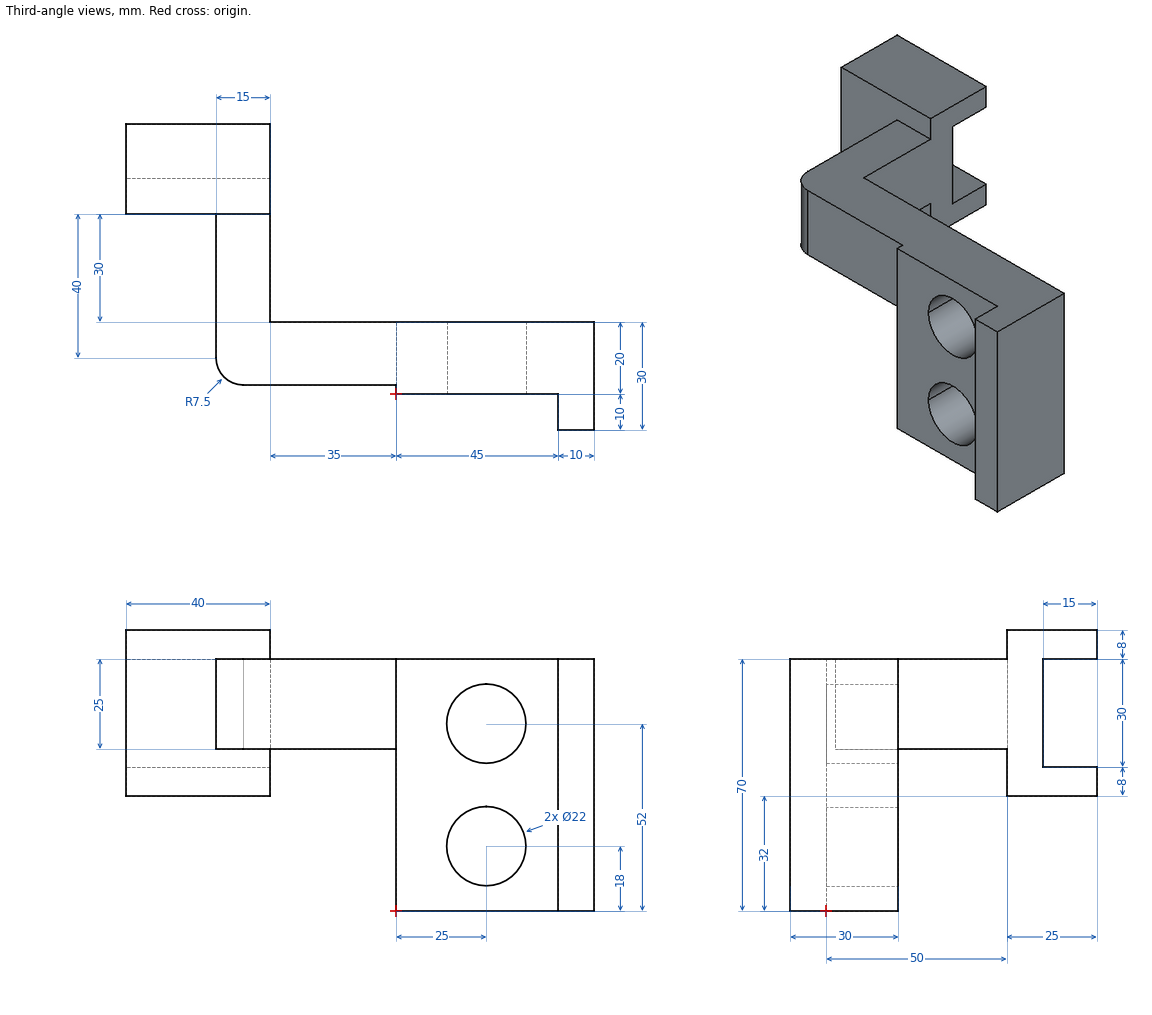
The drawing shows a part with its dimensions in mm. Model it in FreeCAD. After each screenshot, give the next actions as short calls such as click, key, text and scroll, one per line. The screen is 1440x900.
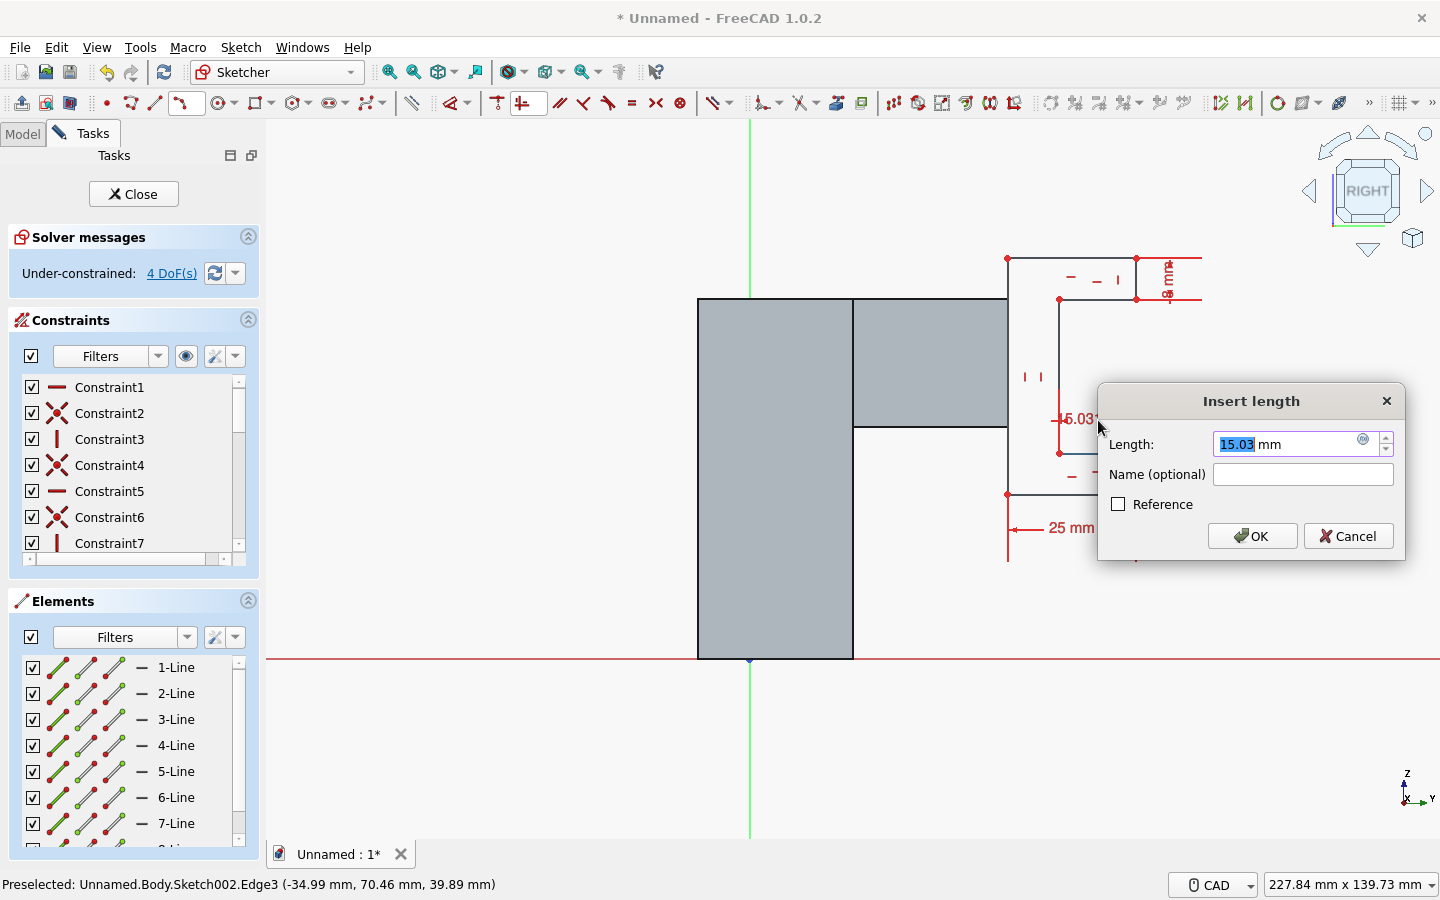
text(15)
key(Return)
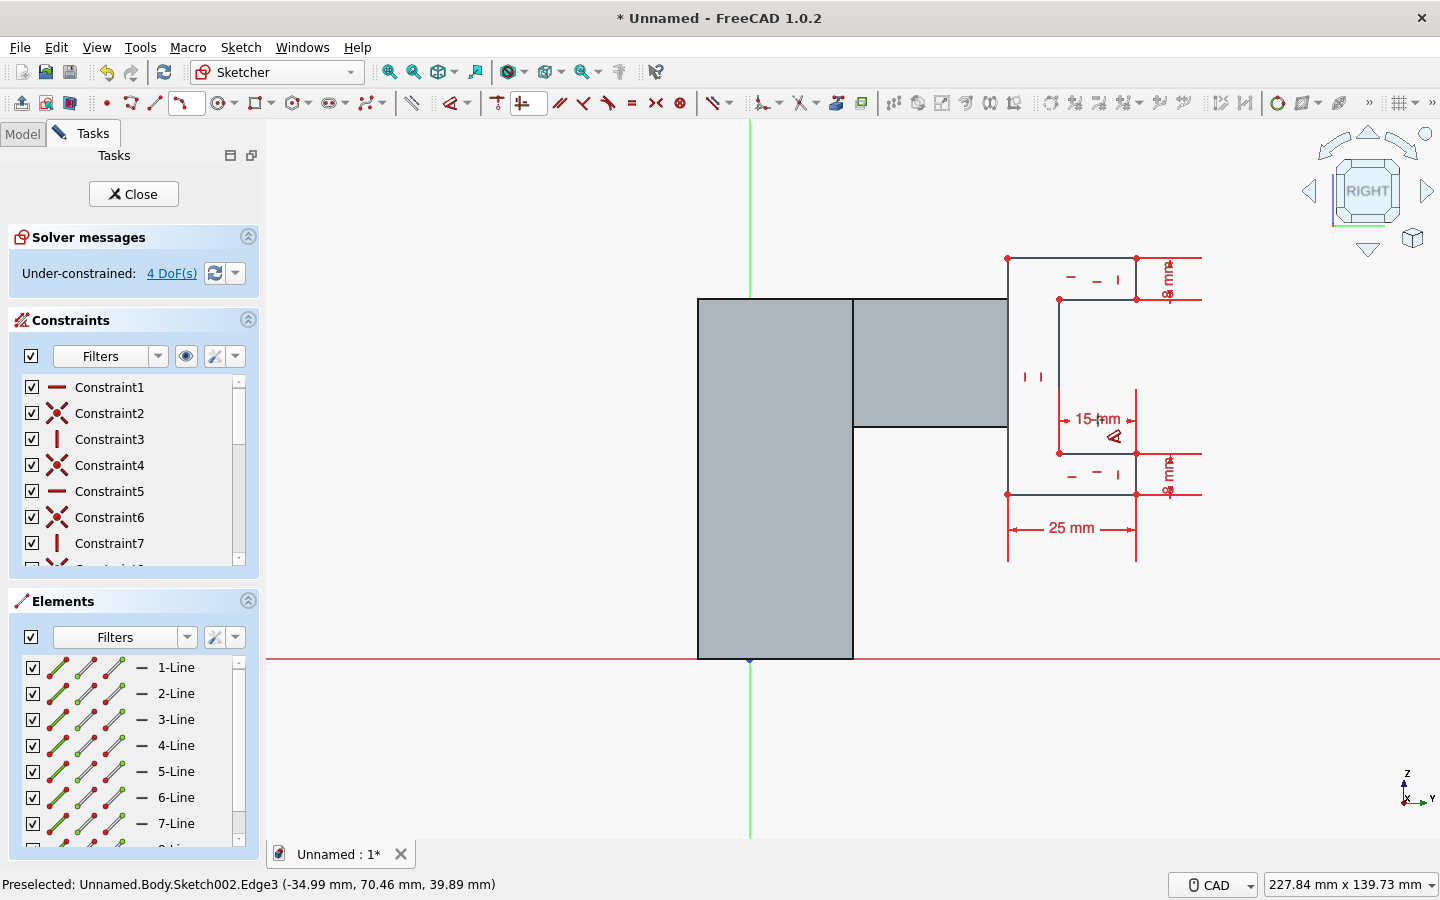
click(1059, 408)
click(1093, 377)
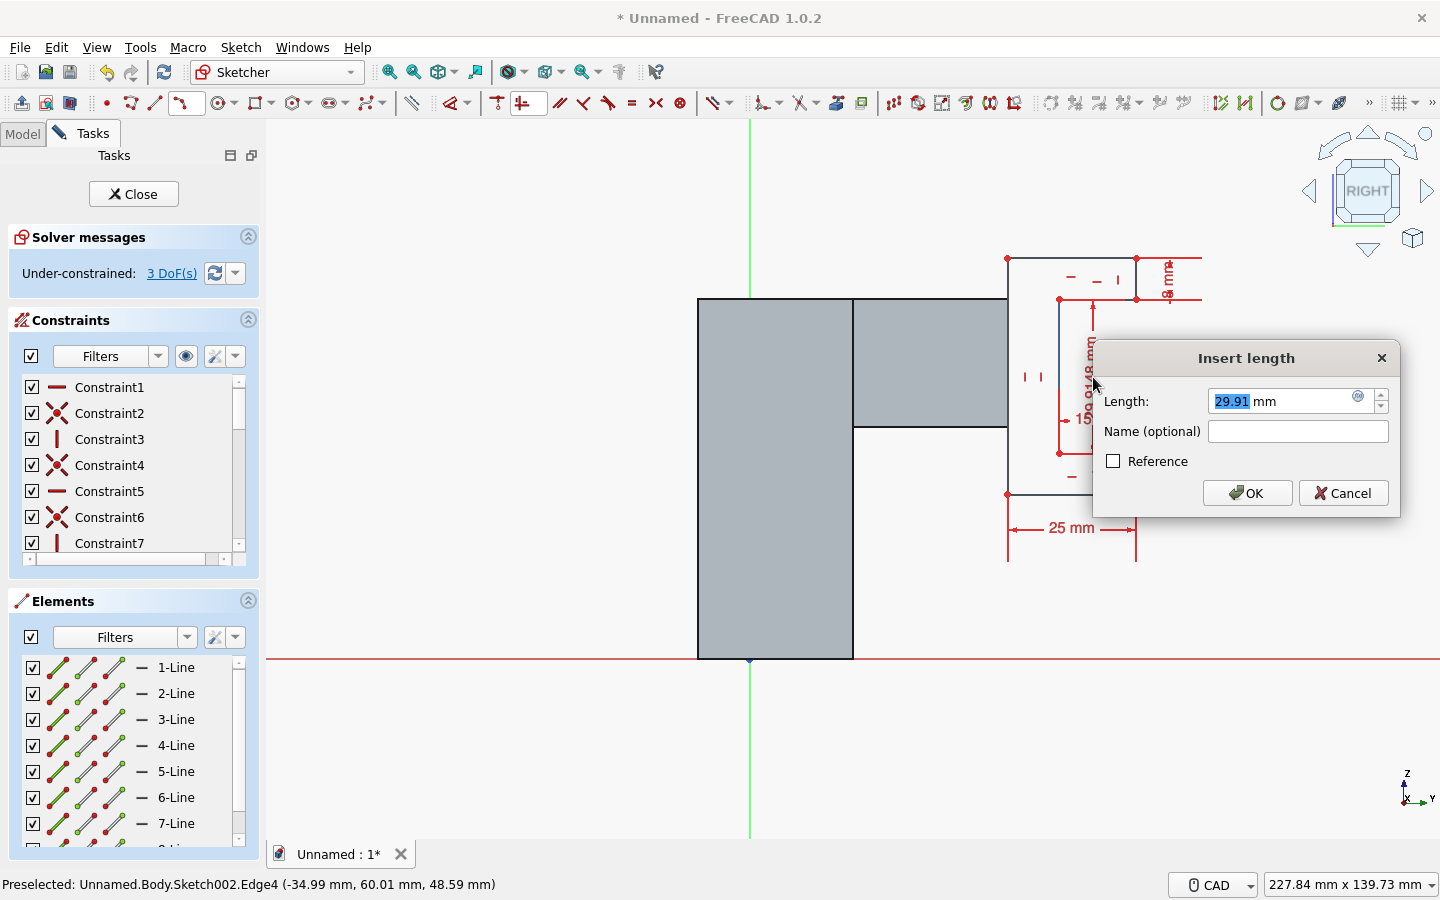
text(30)
key(Return)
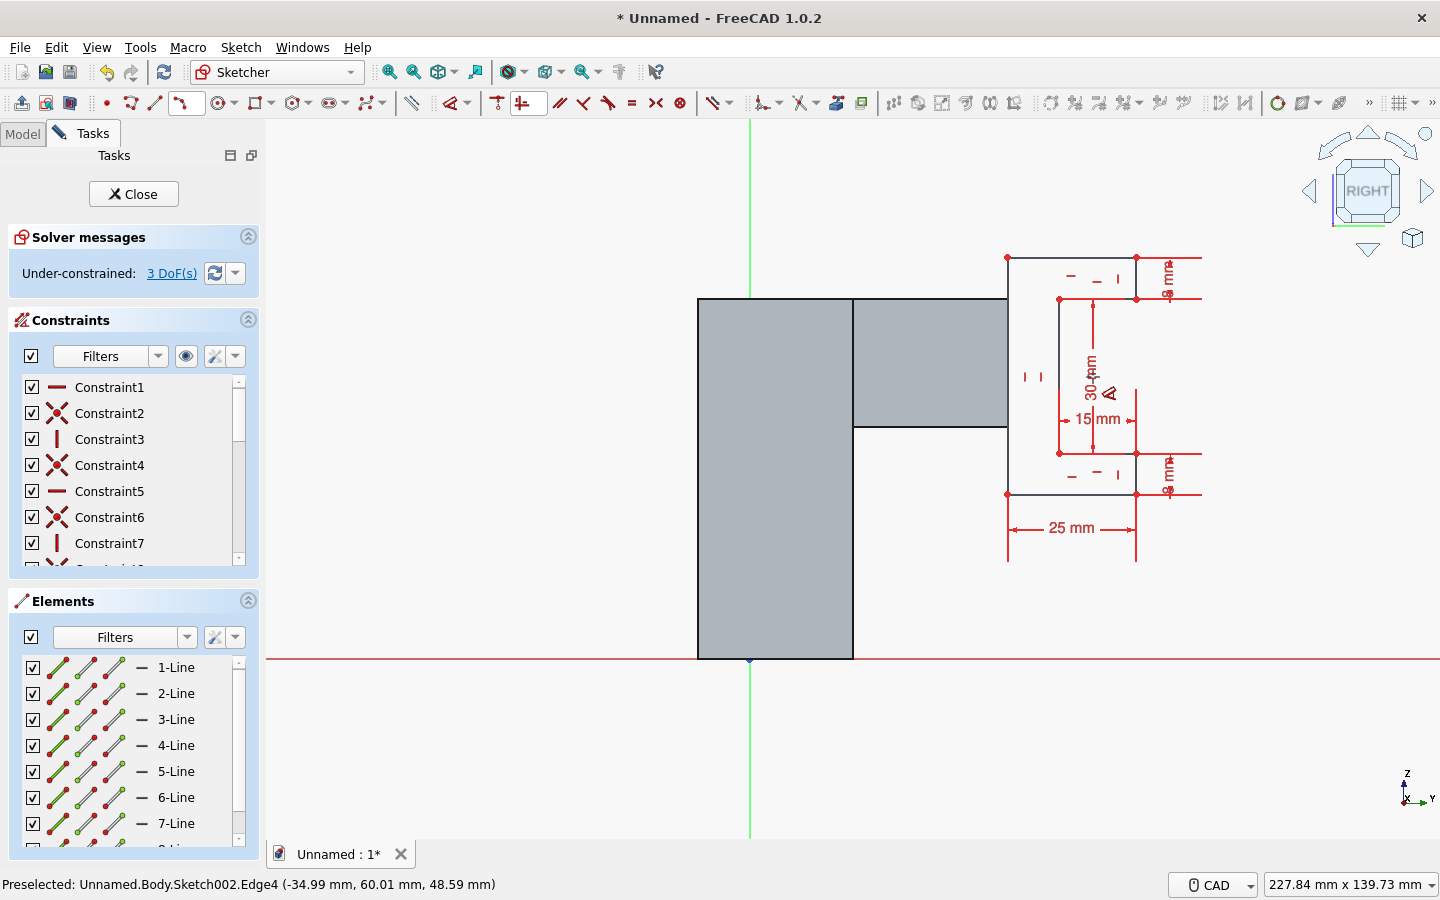
click(1082, 299)
click(1098, 333)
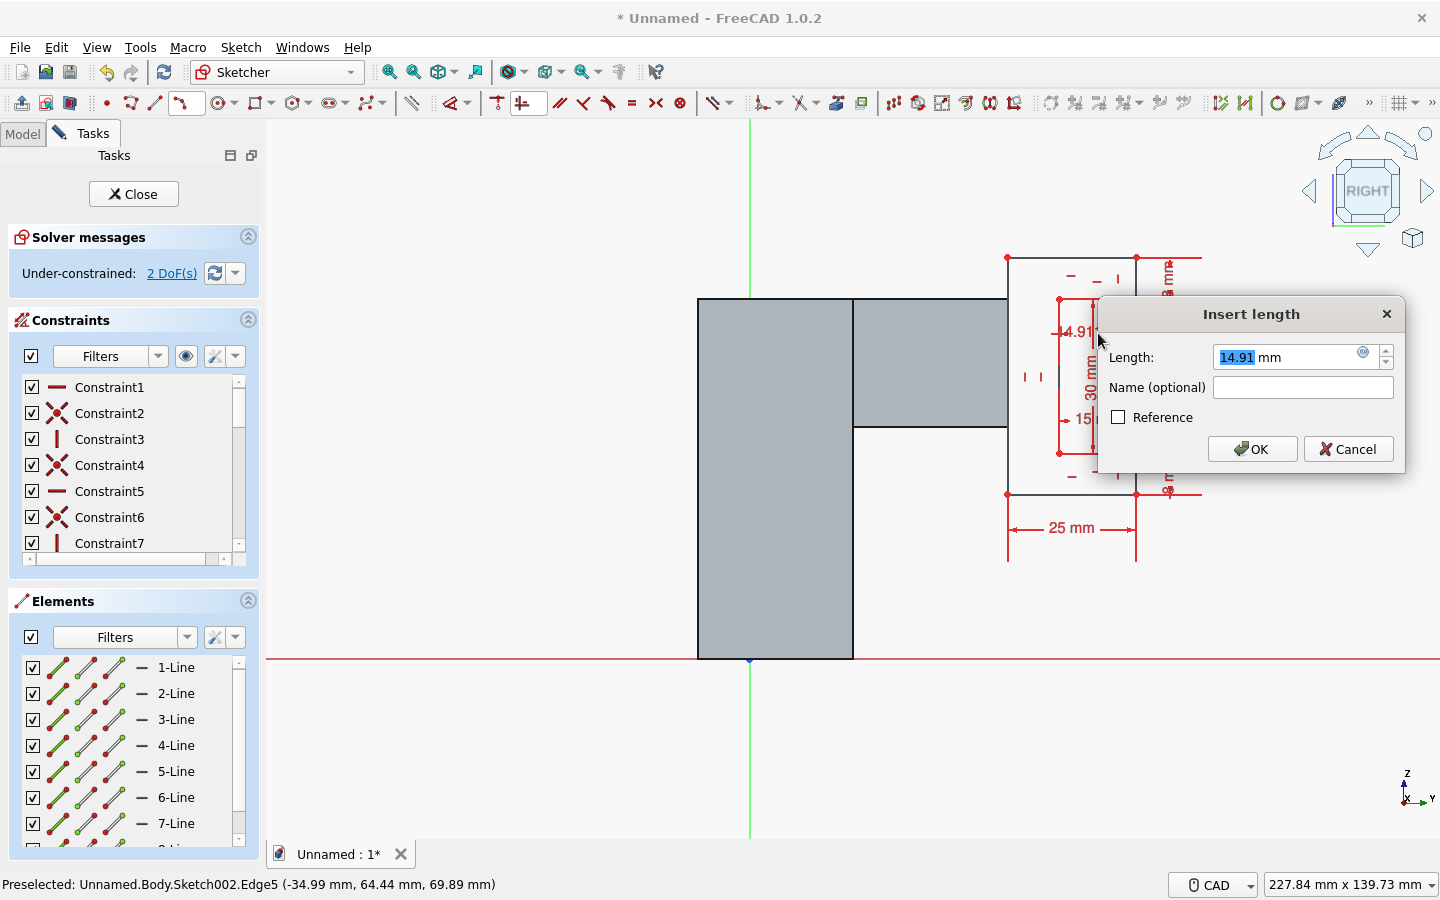
text(15)
key(Return)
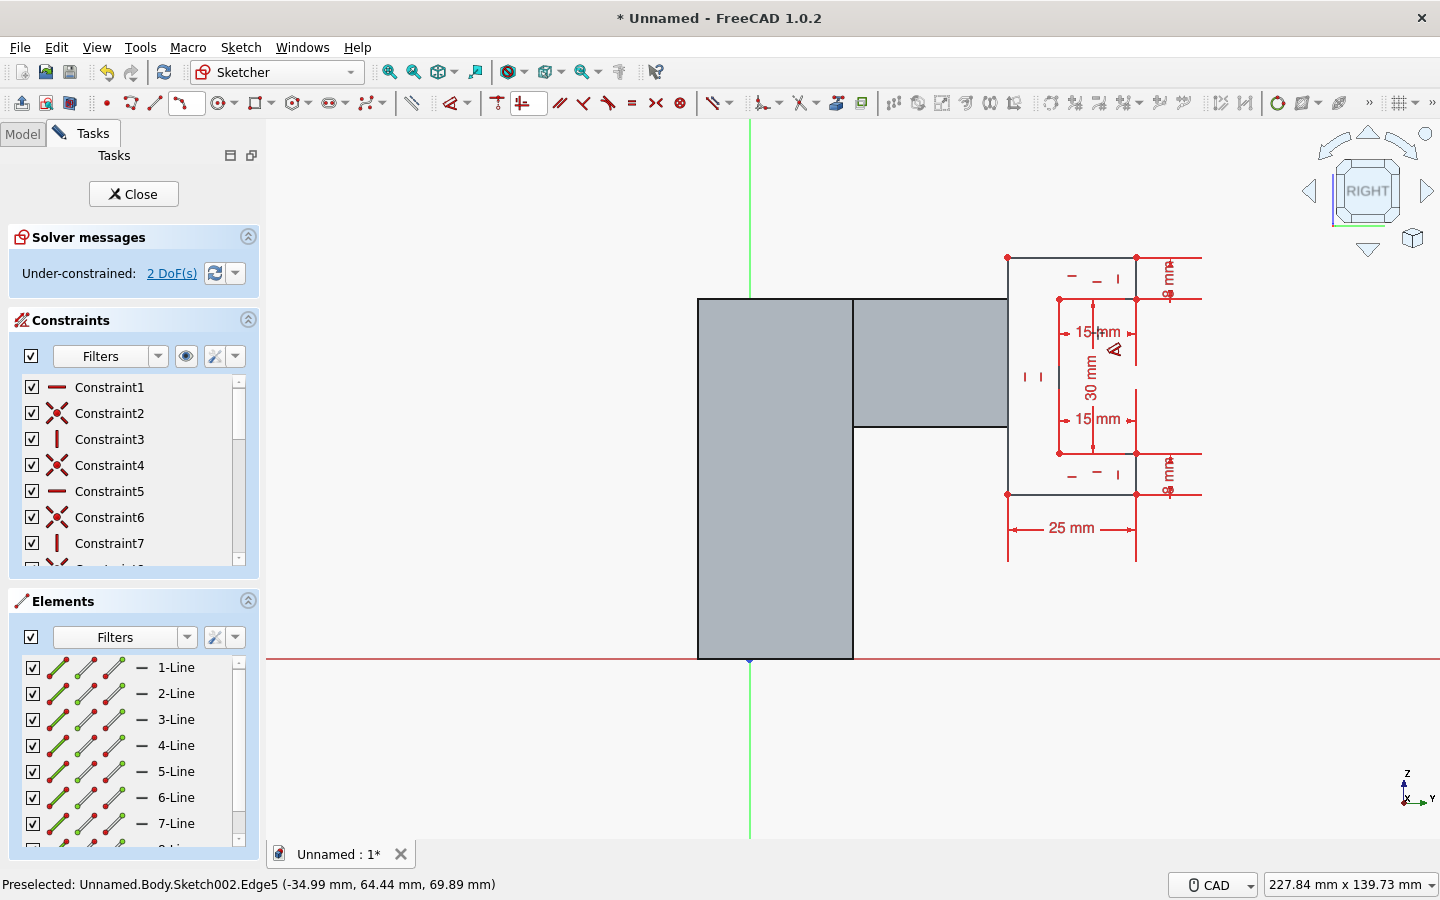
click(1008, 495)
click(879, 693)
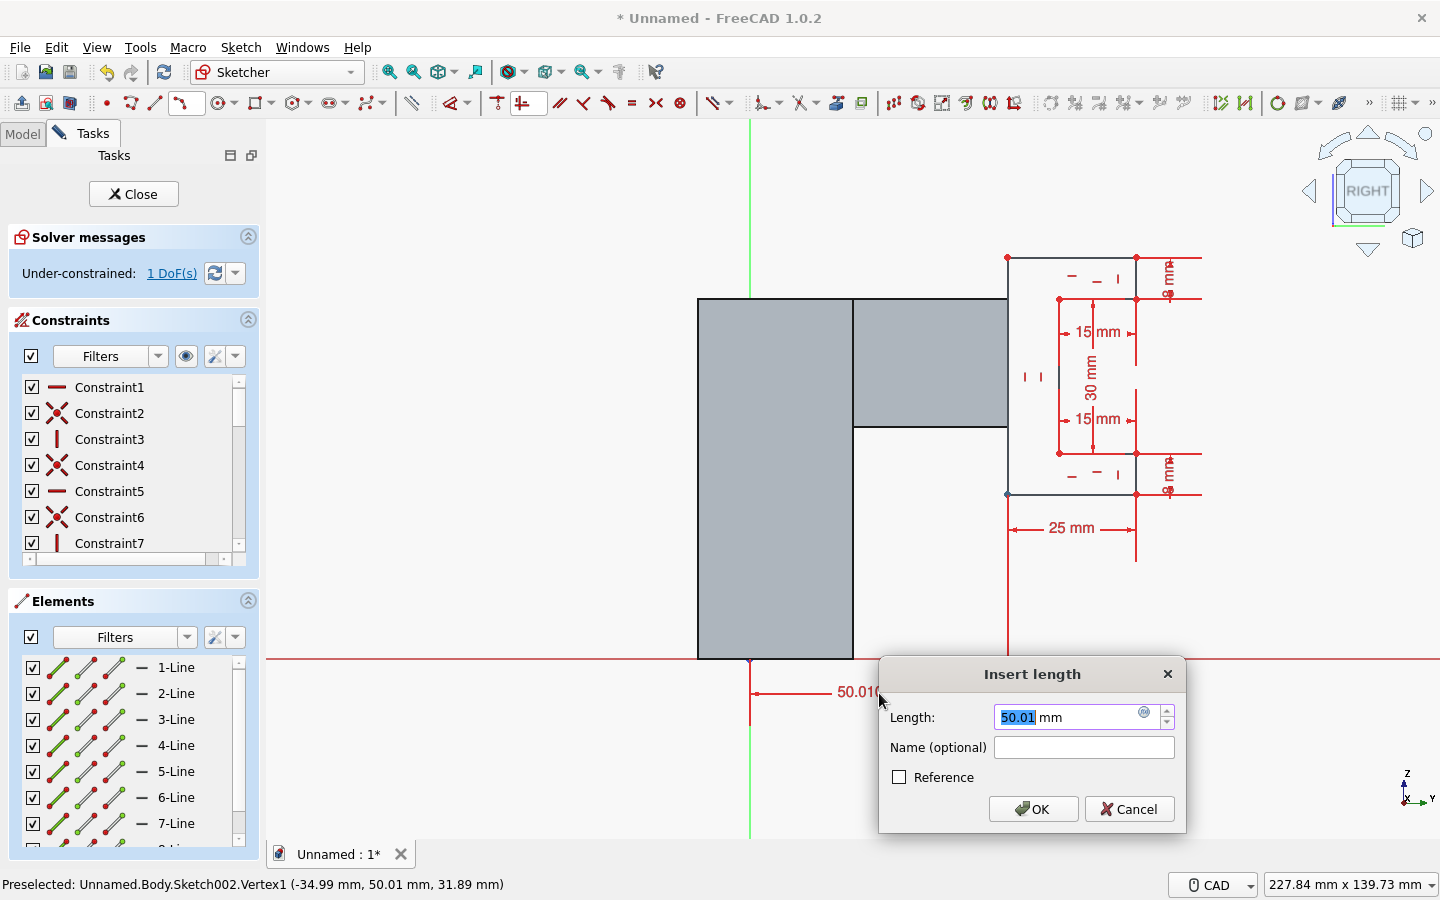
text(50)
key(Return)